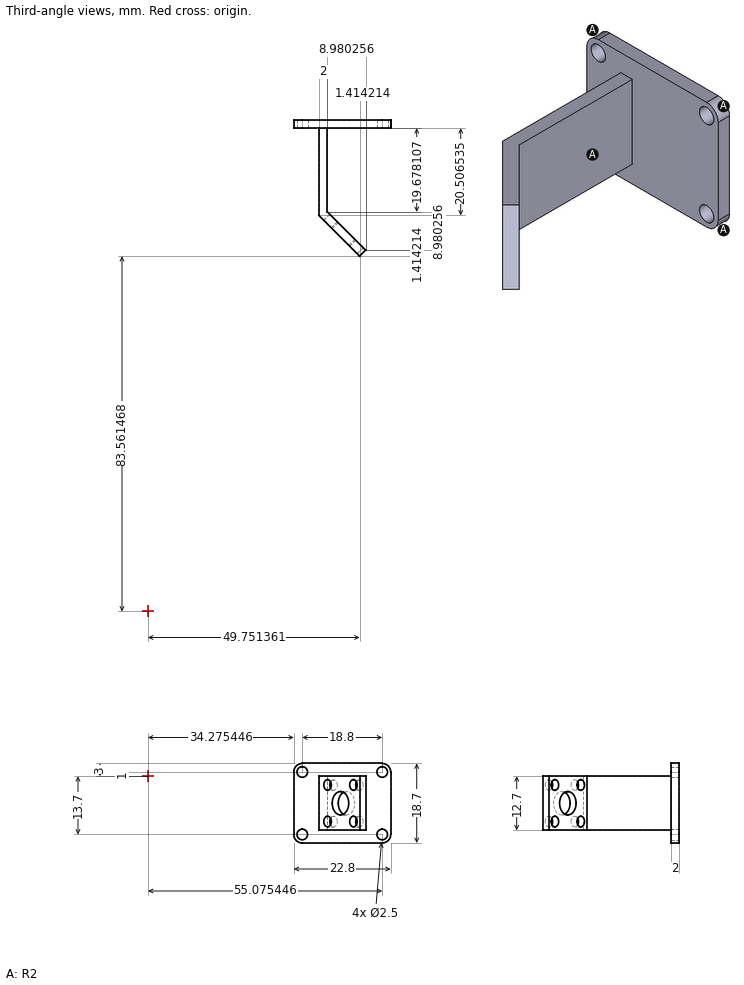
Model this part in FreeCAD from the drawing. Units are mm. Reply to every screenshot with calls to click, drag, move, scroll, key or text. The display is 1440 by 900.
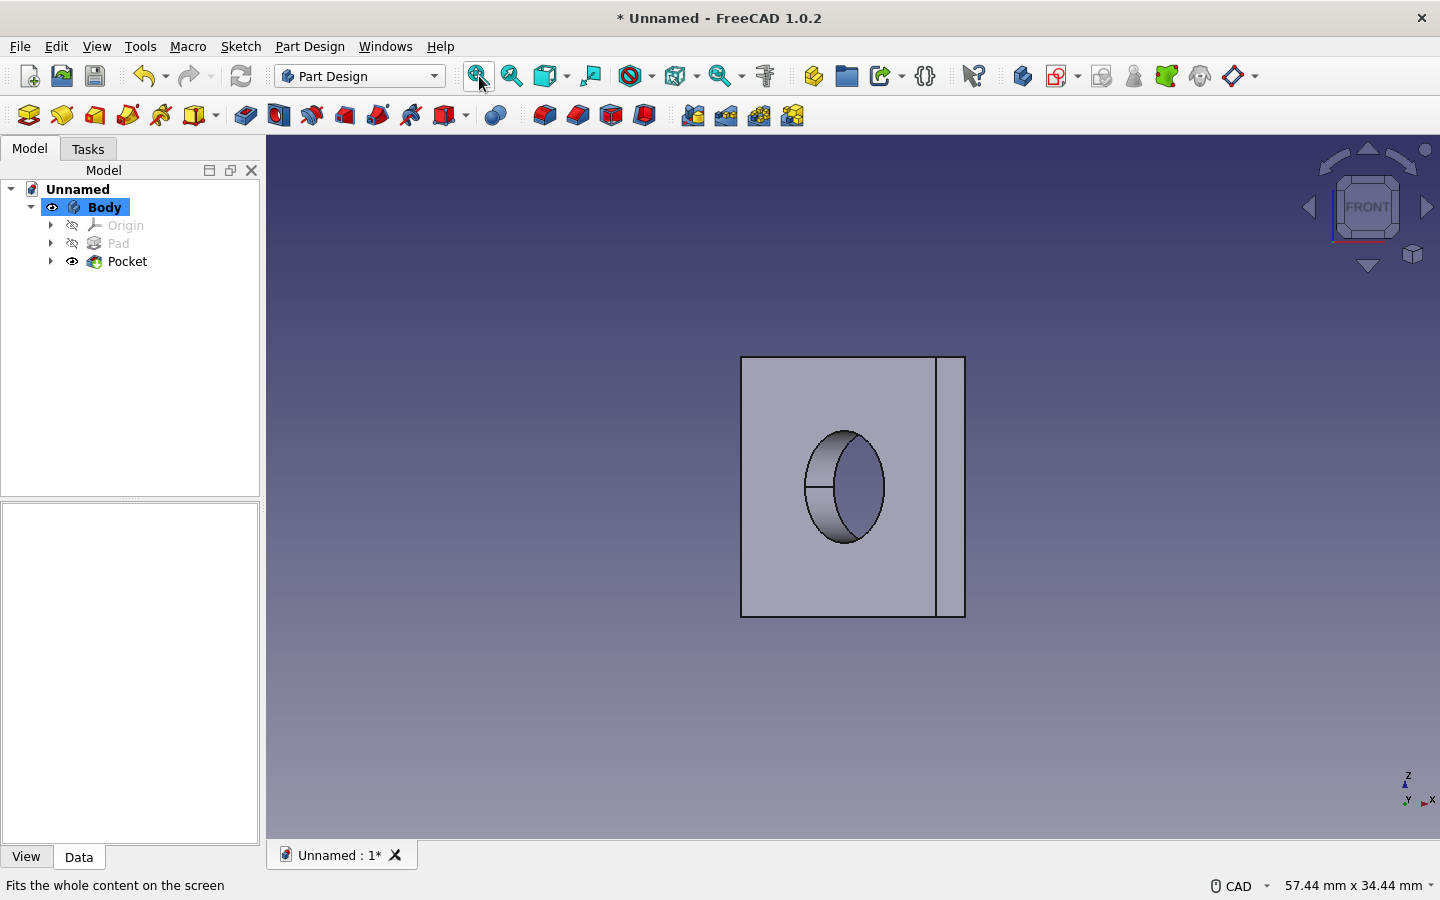
click(479, 76)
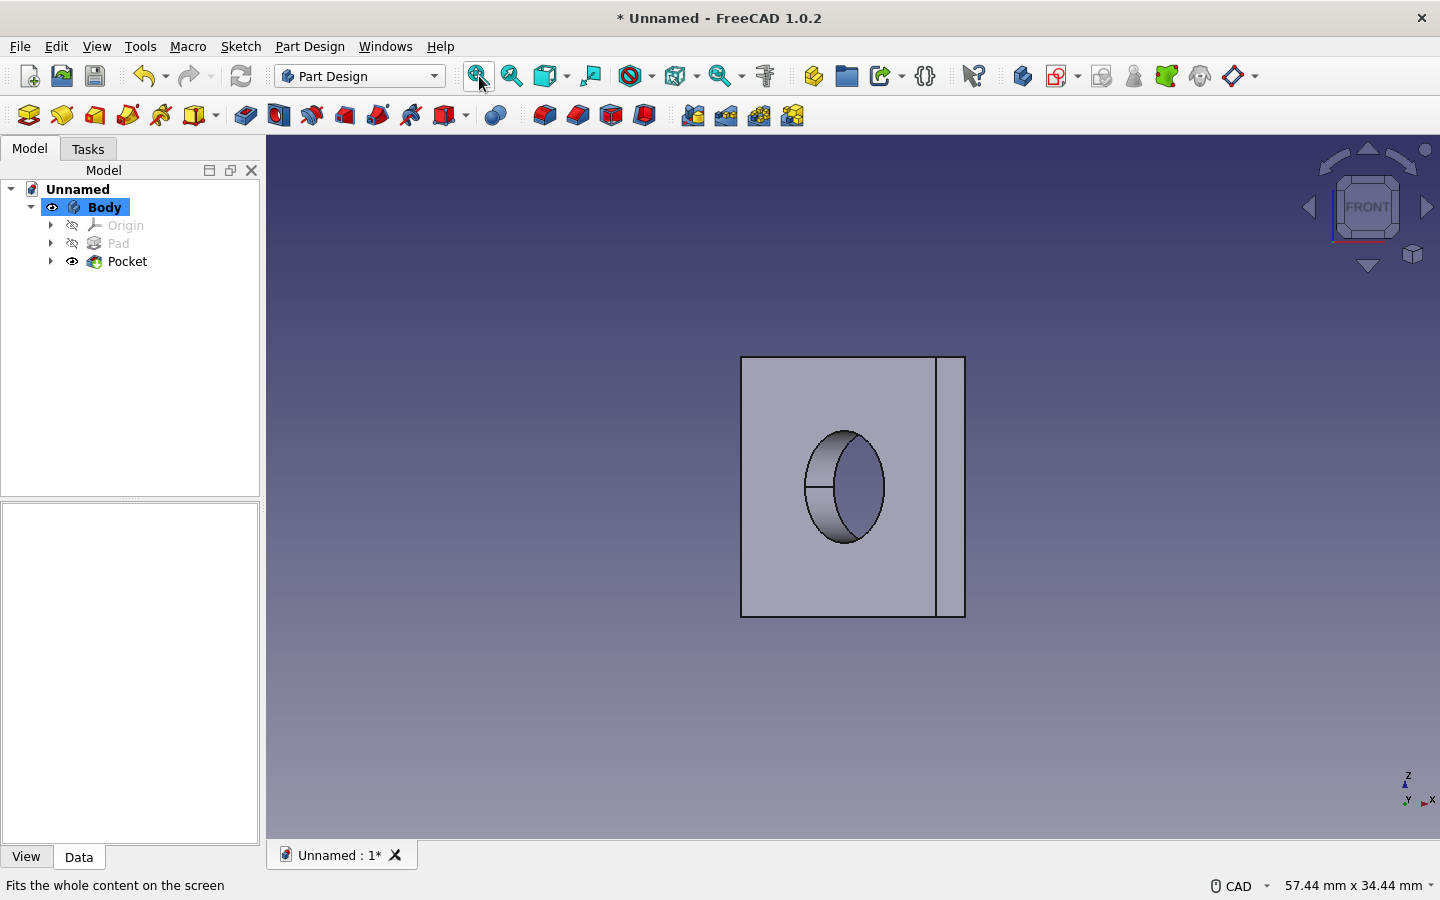
click(783, 412)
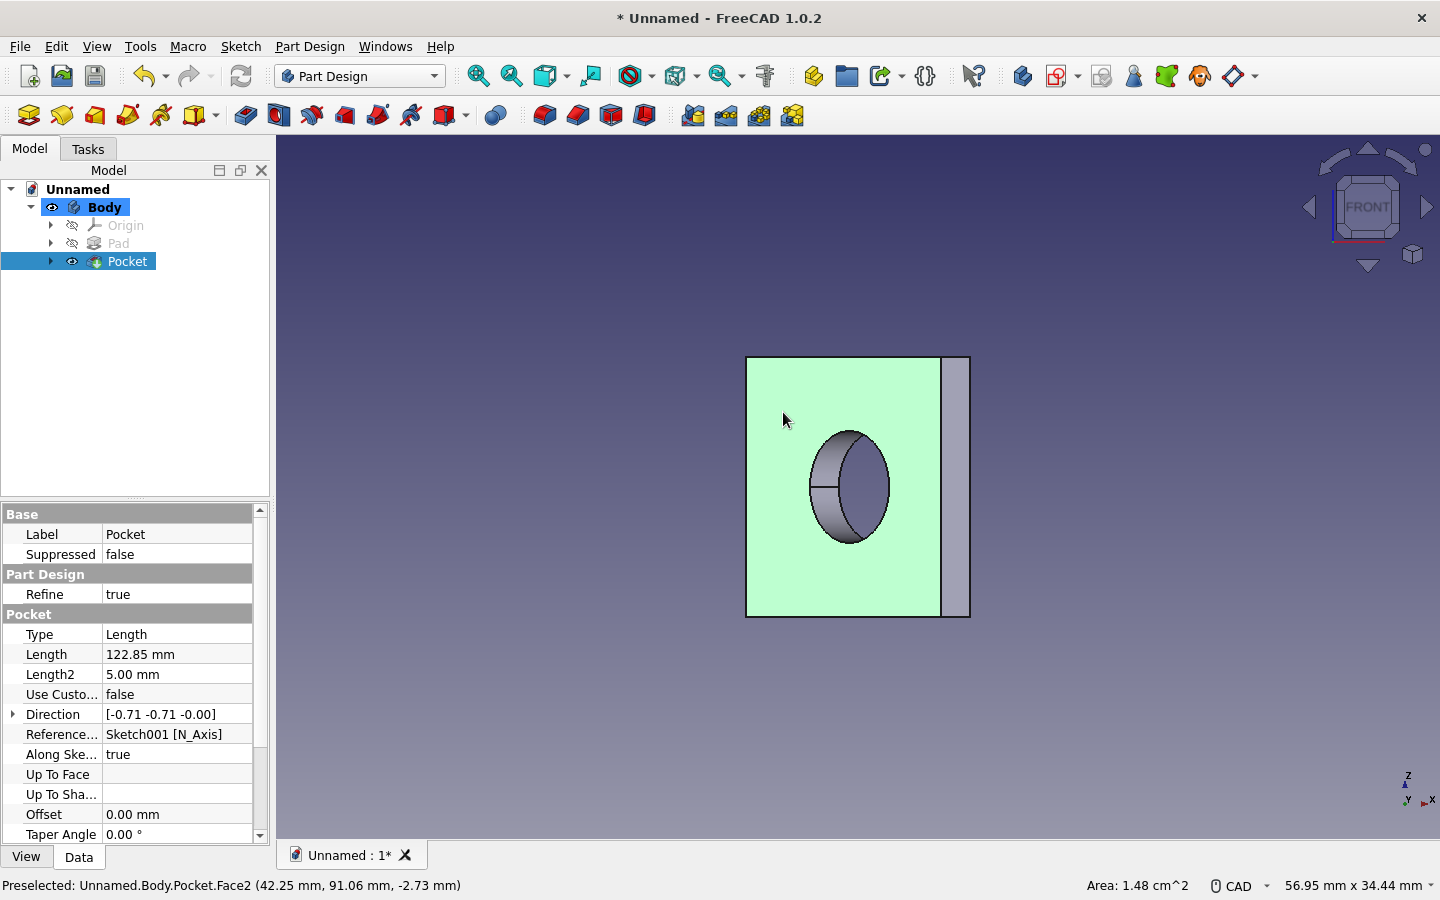
click(1056, 76)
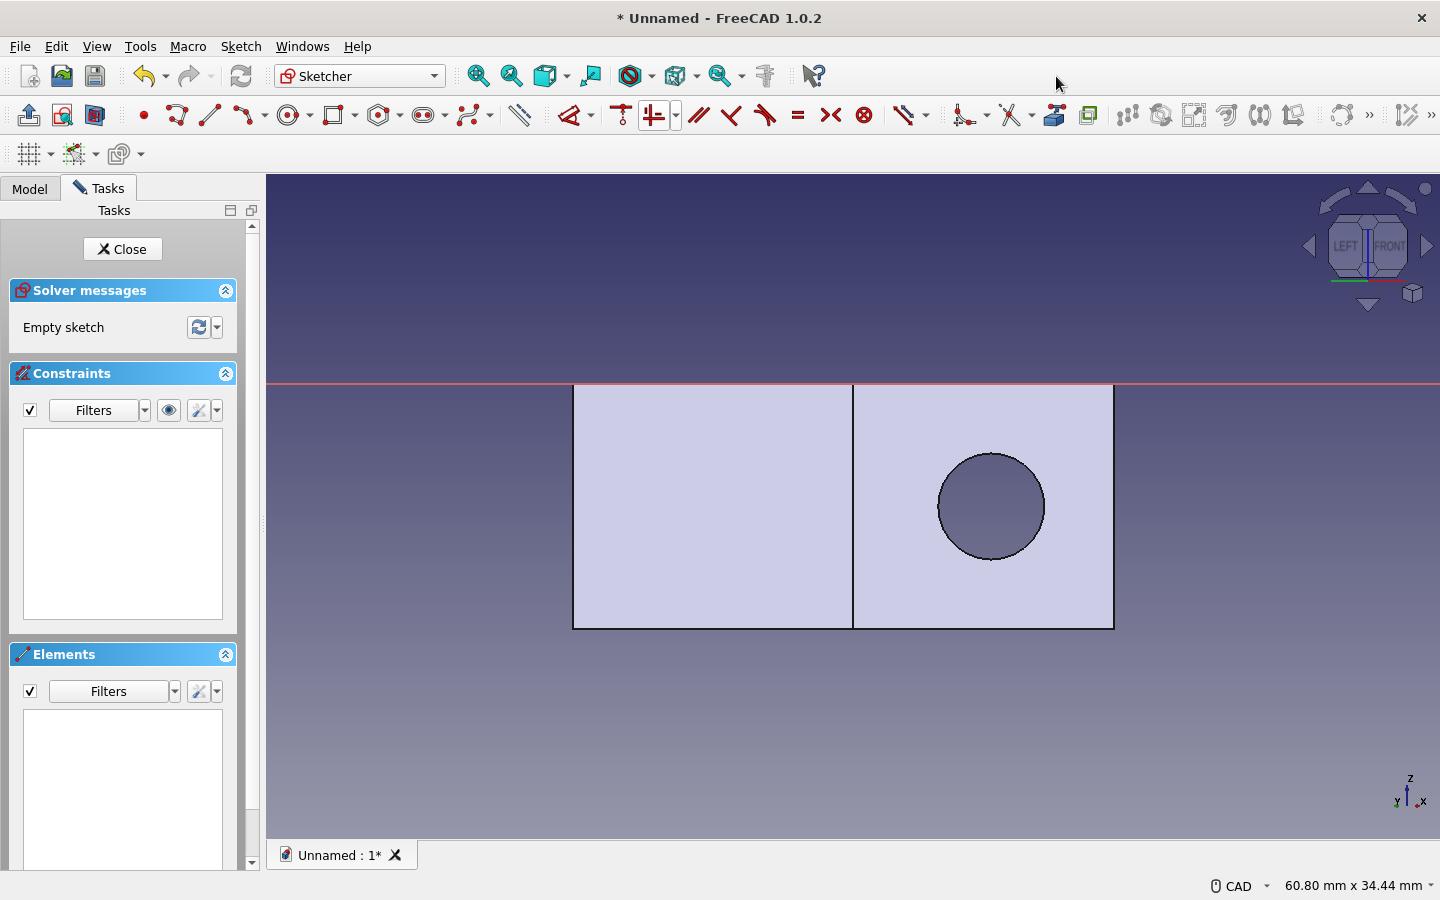
click(95, 116)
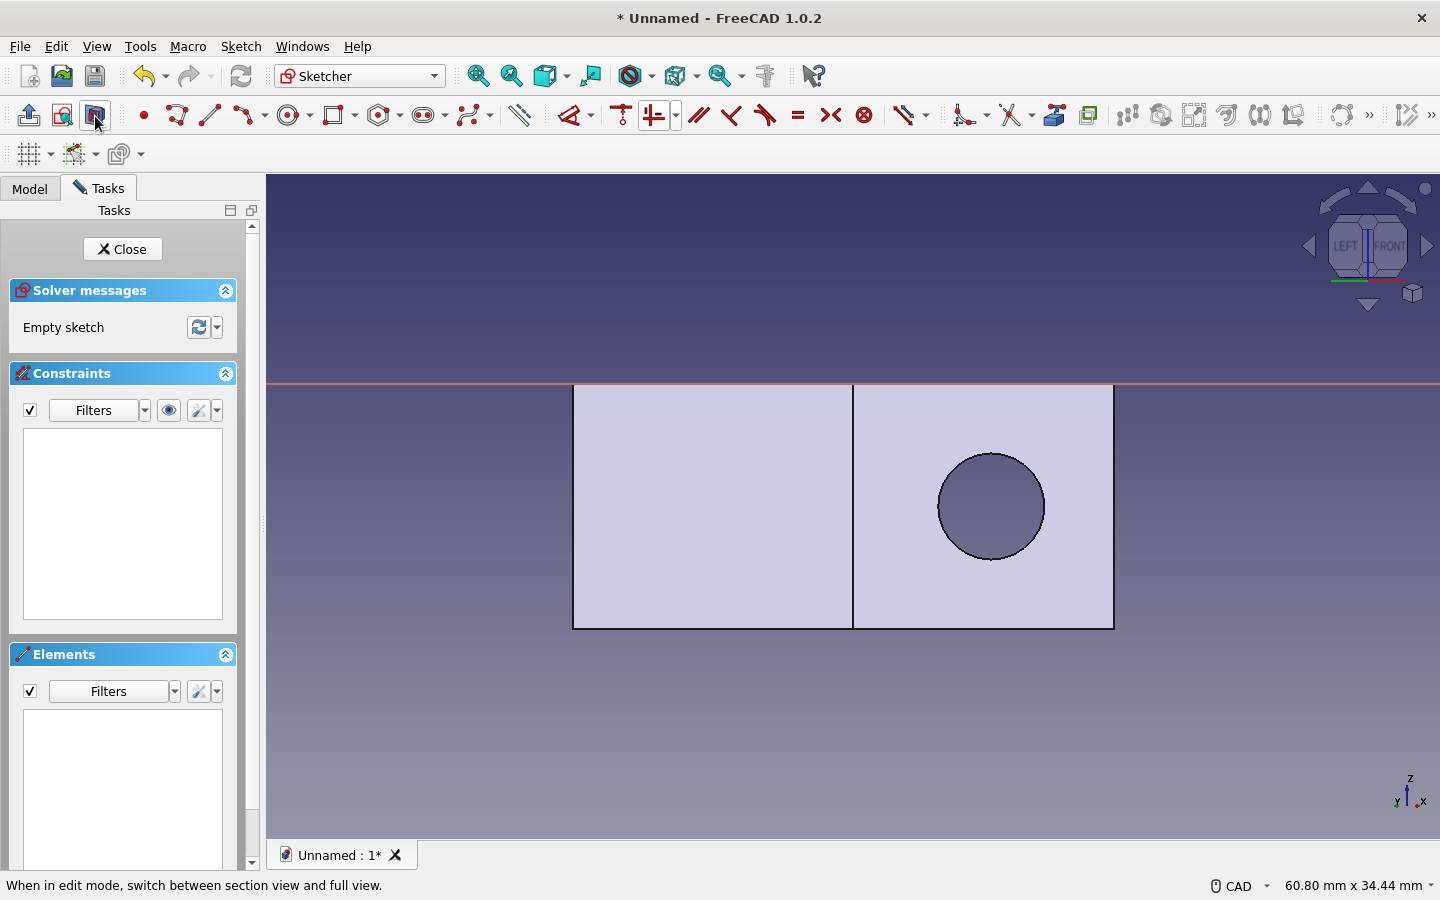
scroll(1243, 506, up, 3)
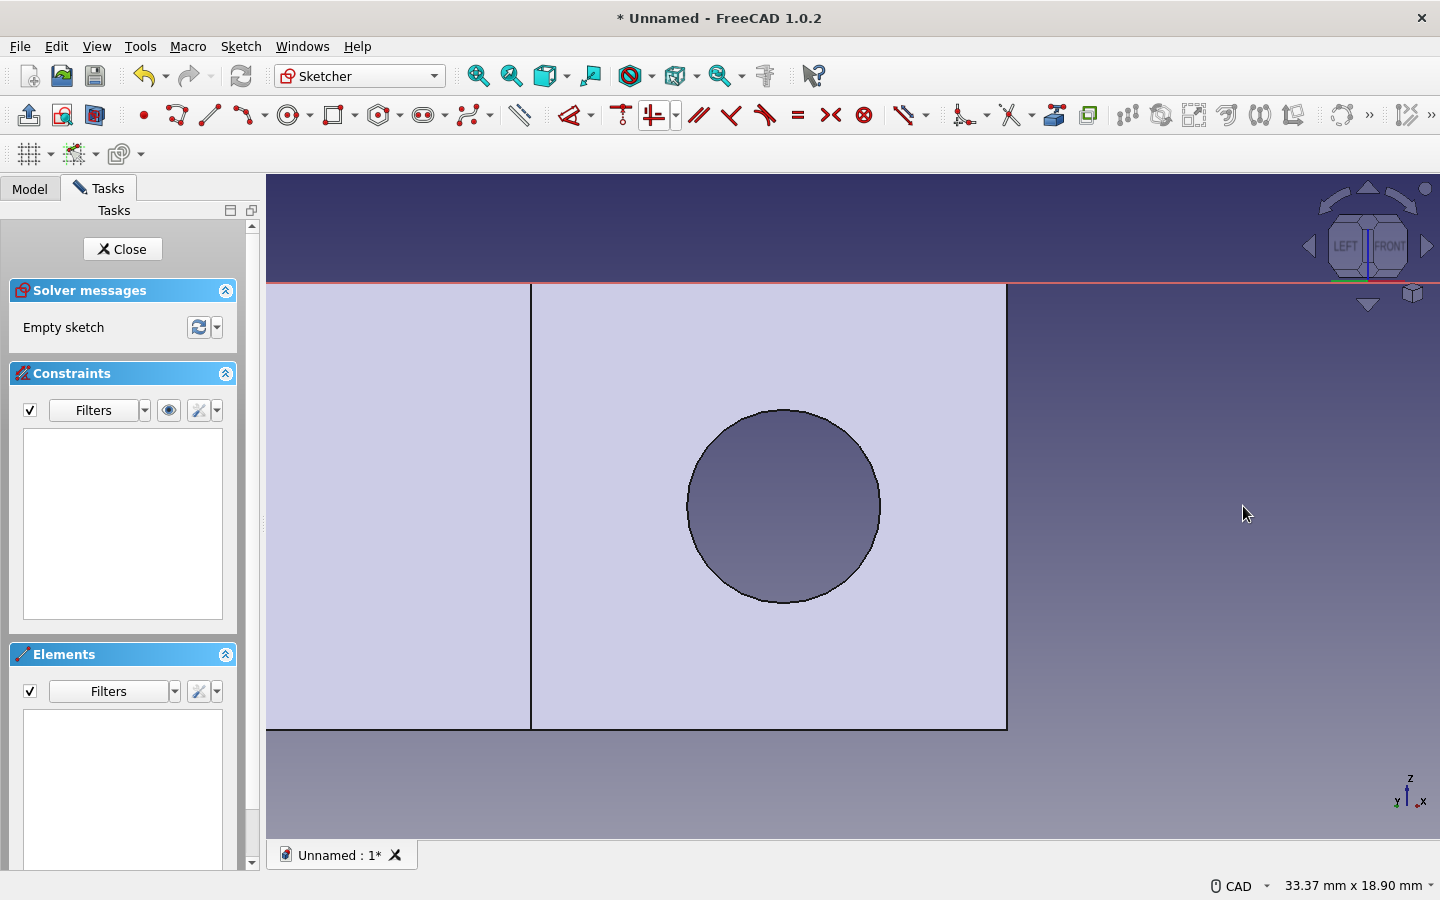
click(288, 116)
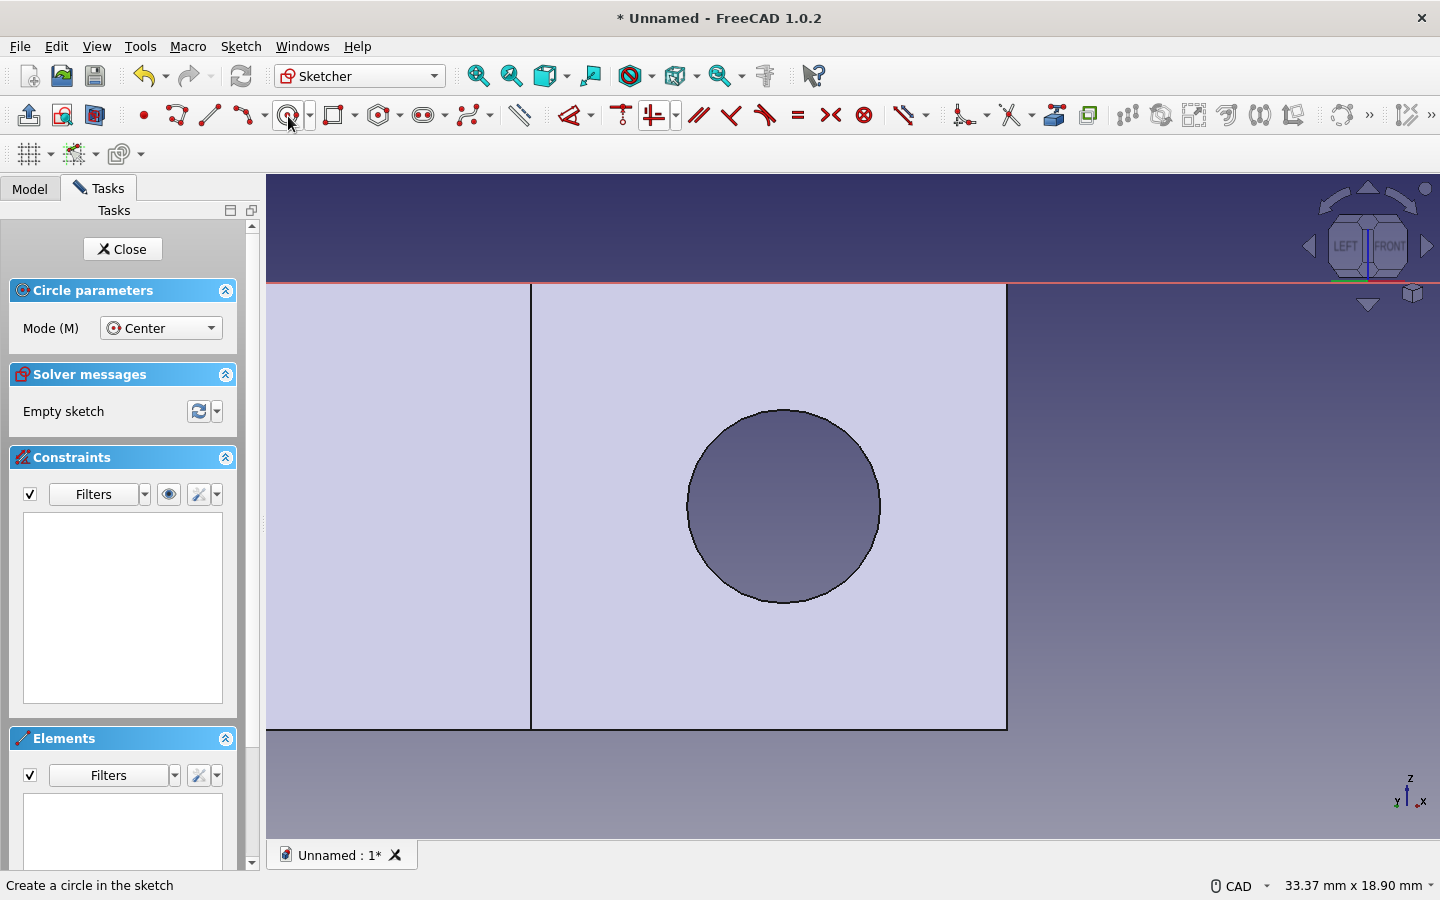
click(632, 658)
move(664, 627)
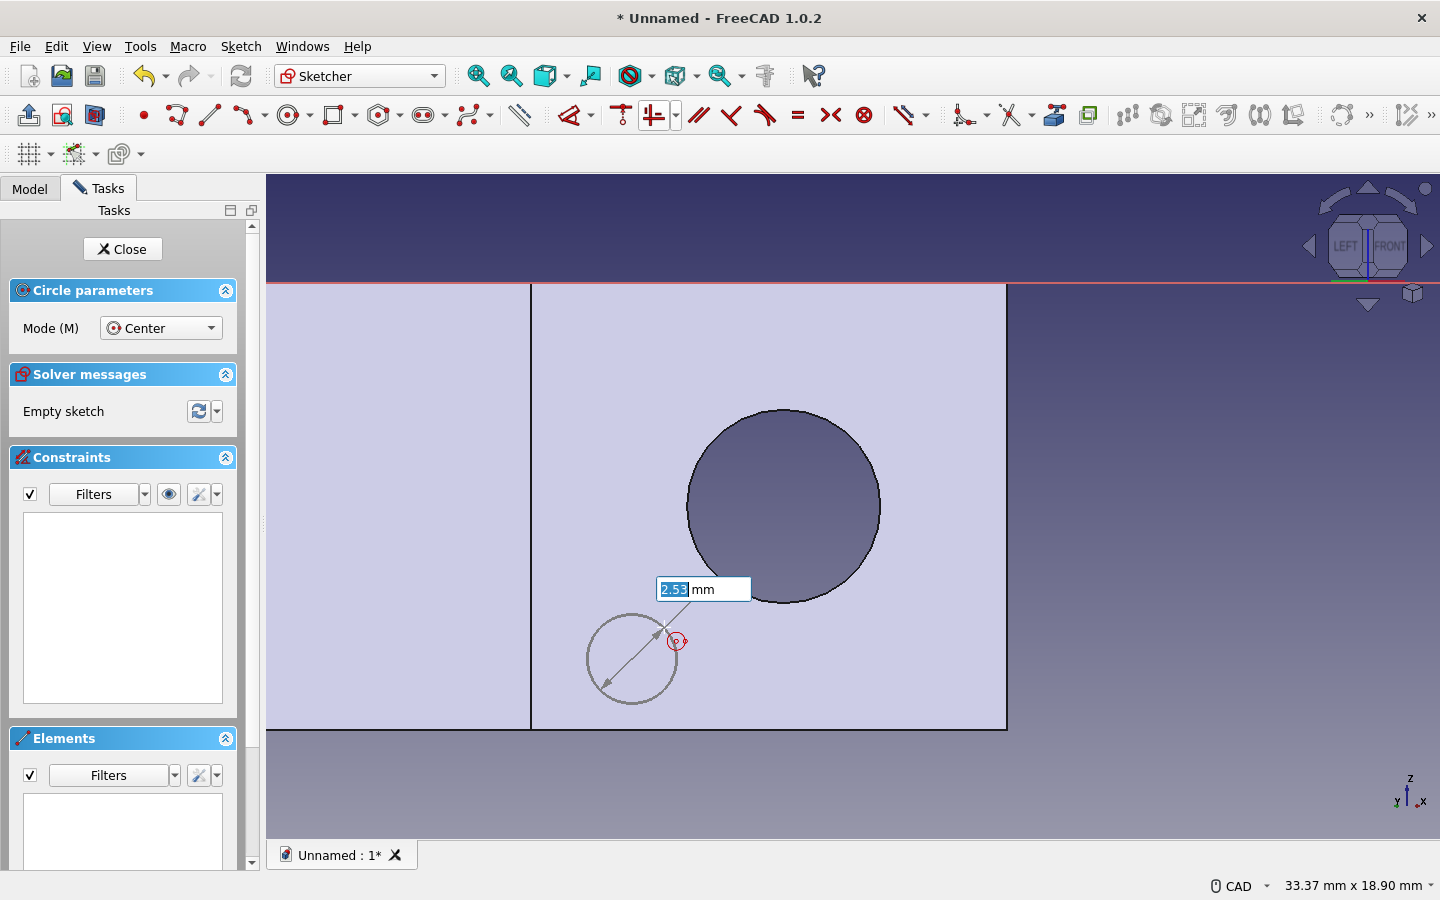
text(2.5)
key(Return)